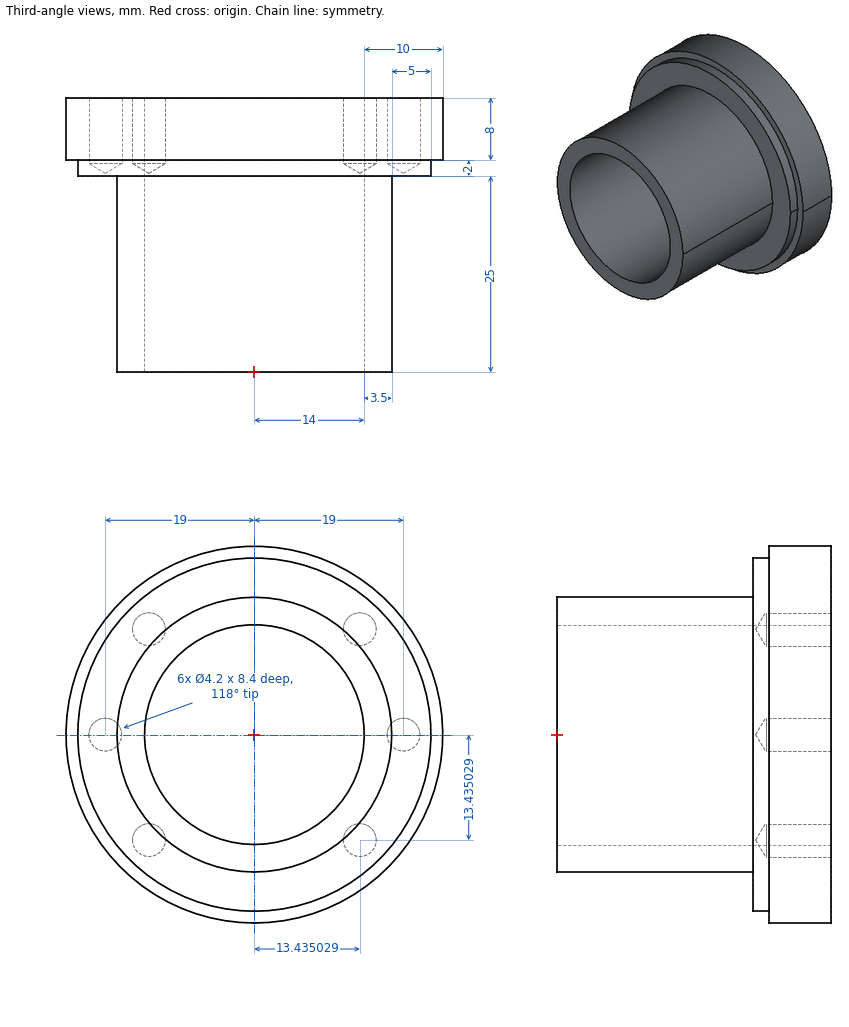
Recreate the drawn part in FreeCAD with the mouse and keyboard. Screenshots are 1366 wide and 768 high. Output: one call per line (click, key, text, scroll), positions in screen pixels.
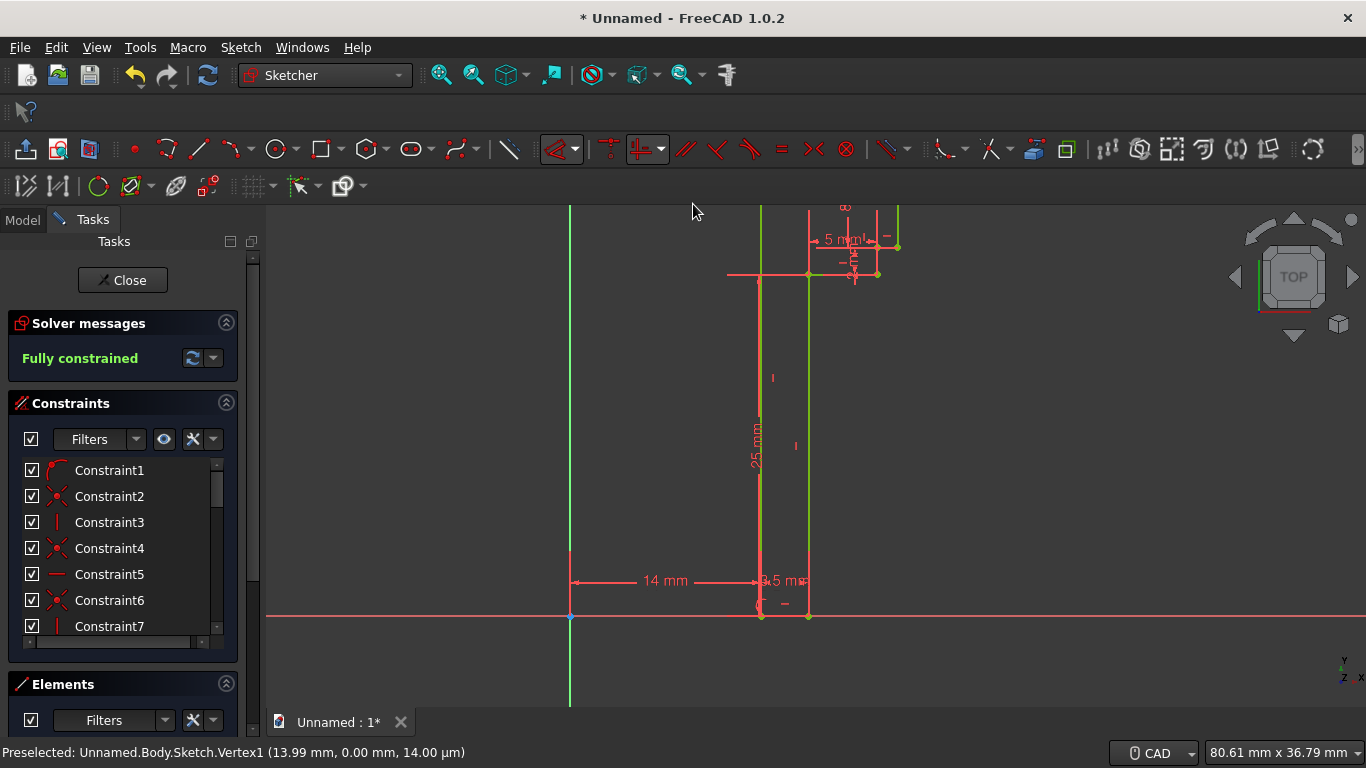
click(123, 280)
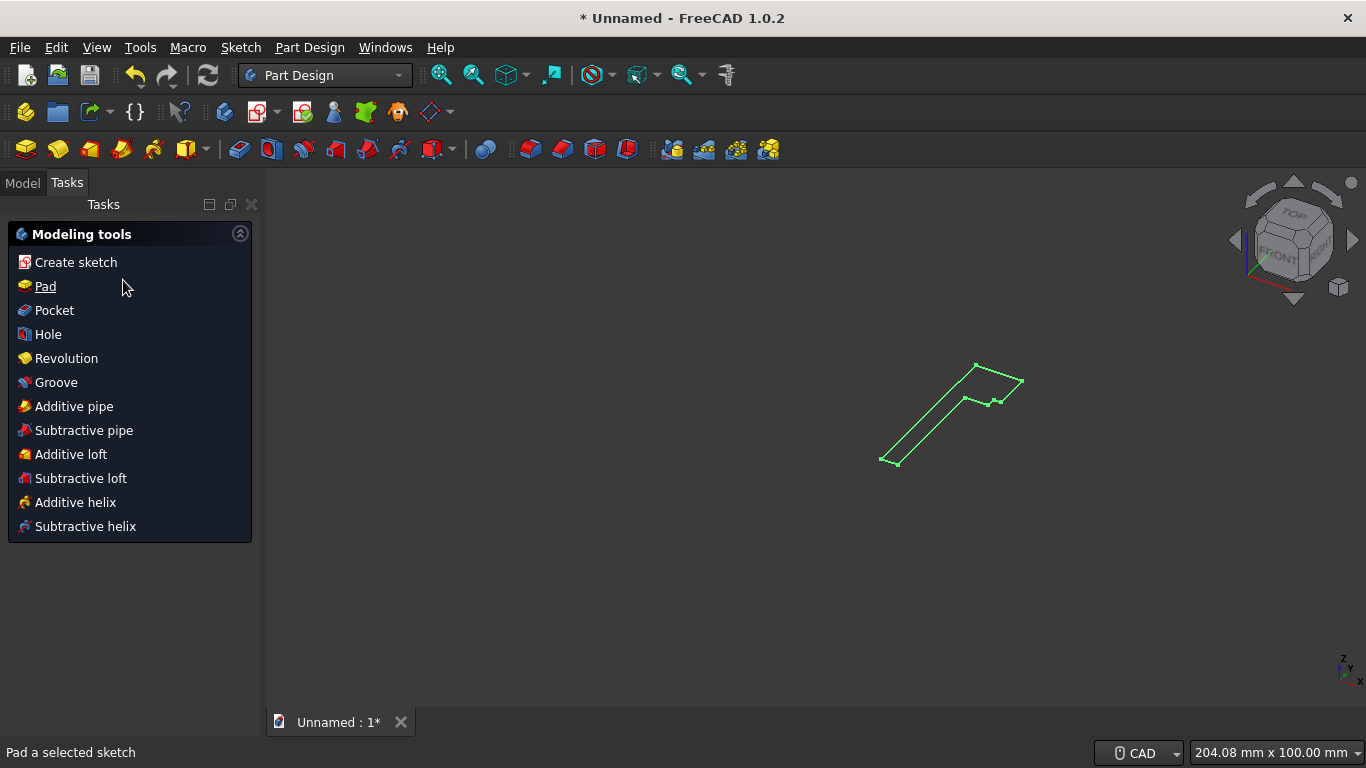
click(58, 150)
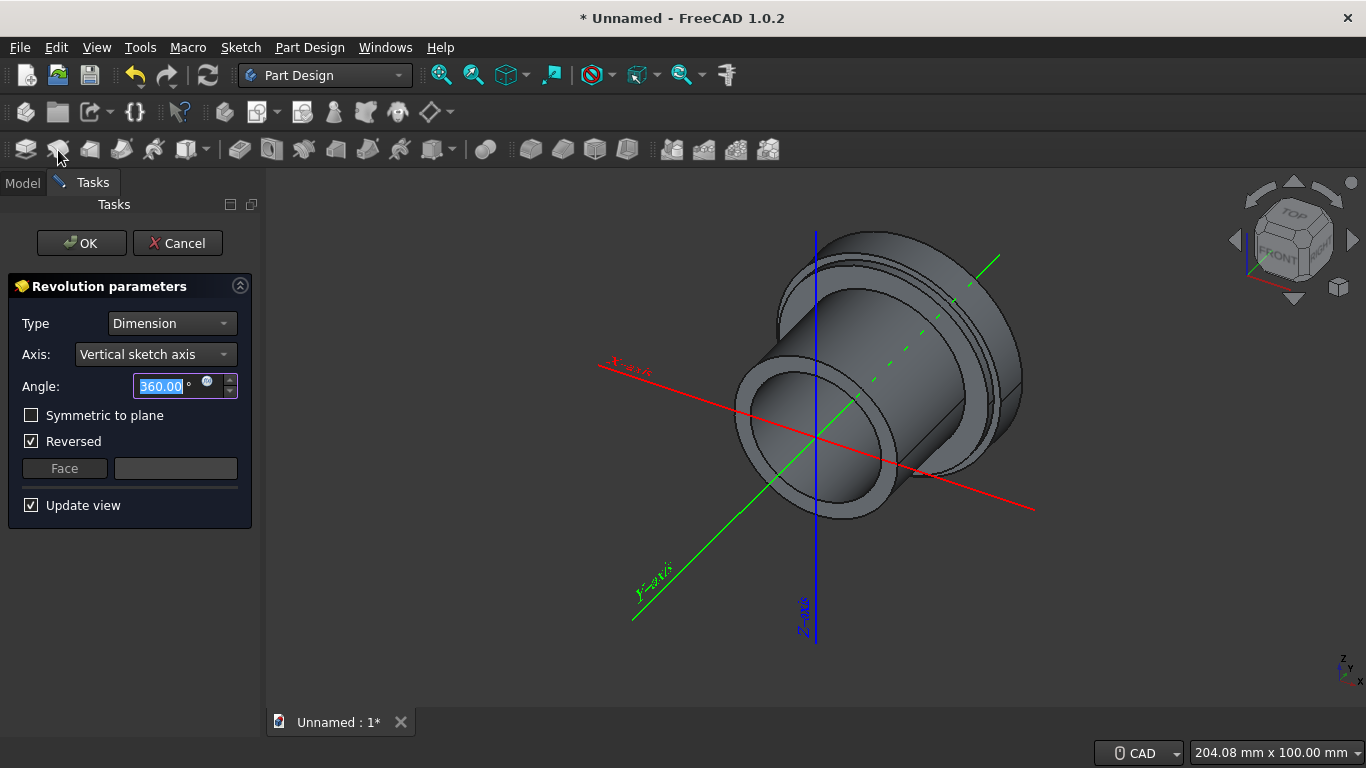
click(82, 243)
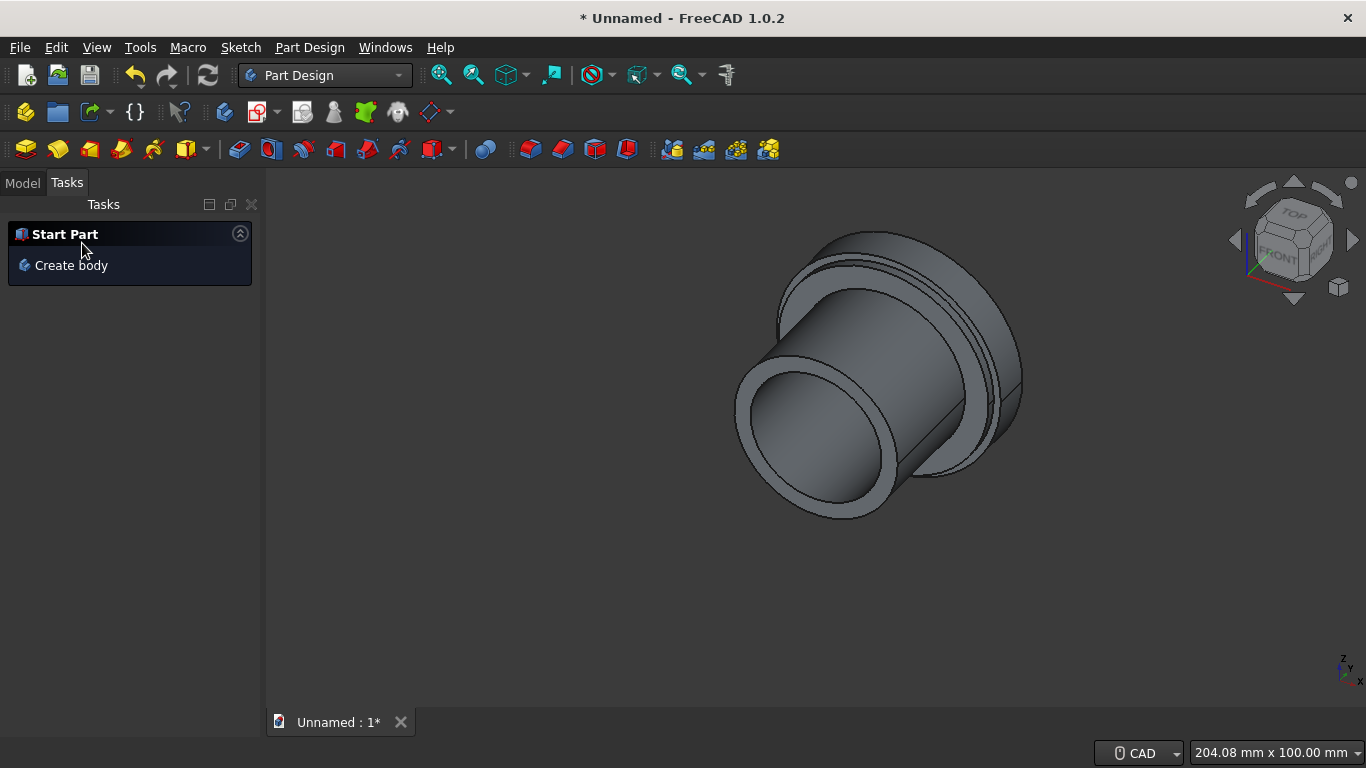
key(4)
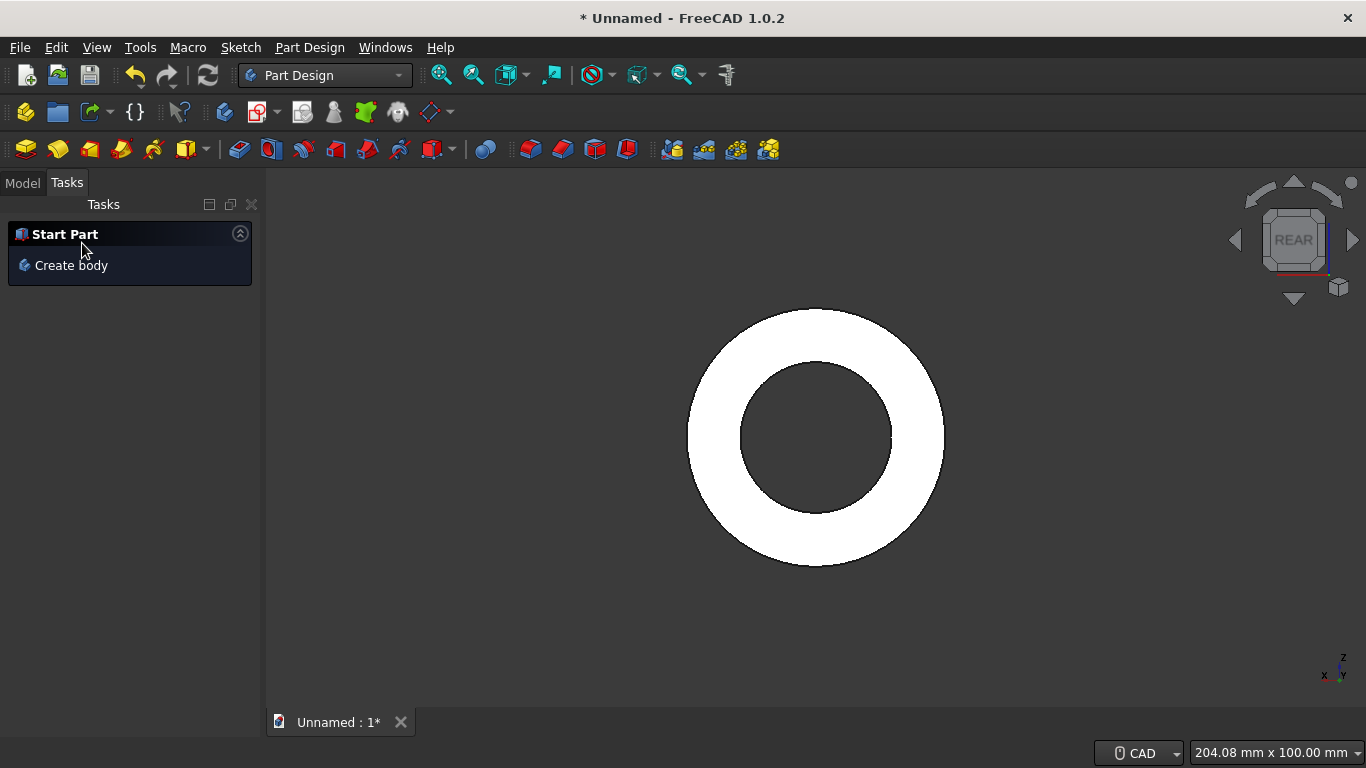
click(890, 510)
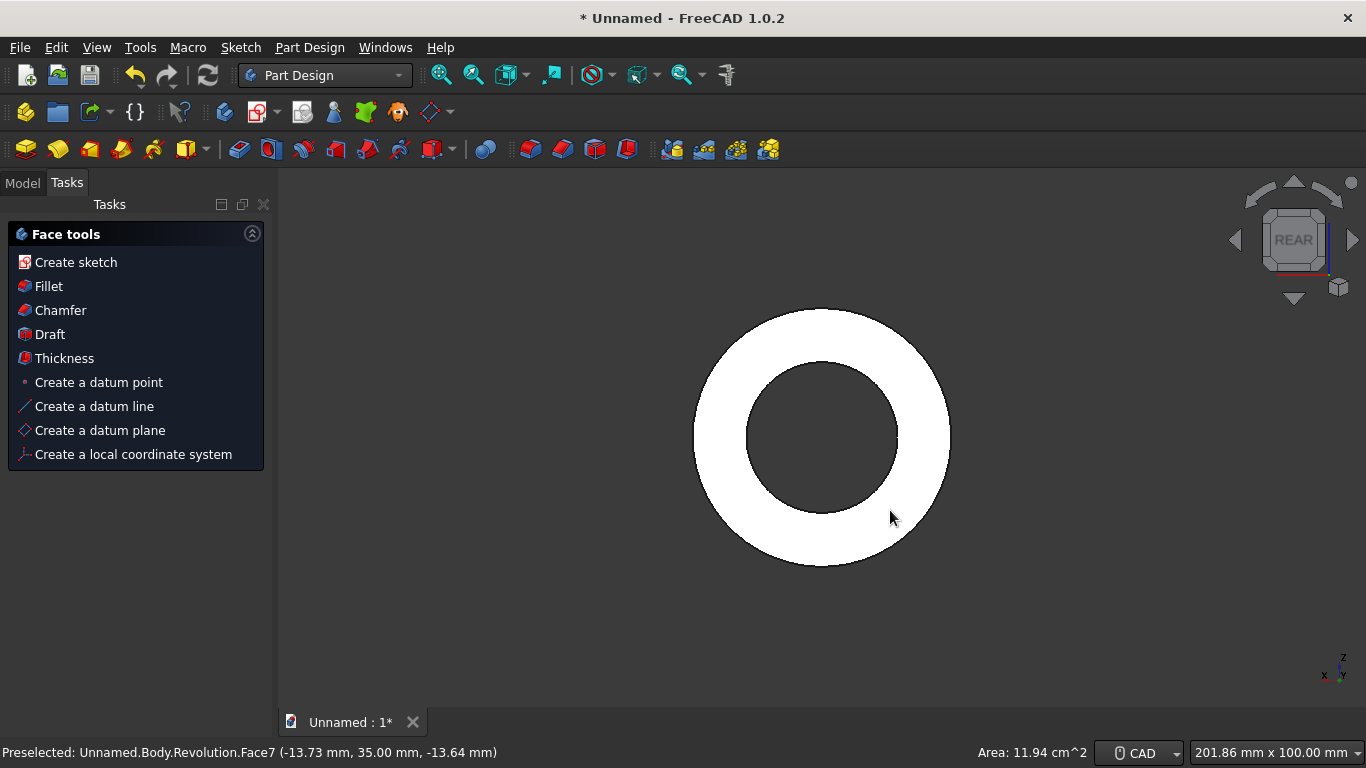
click(258, 112)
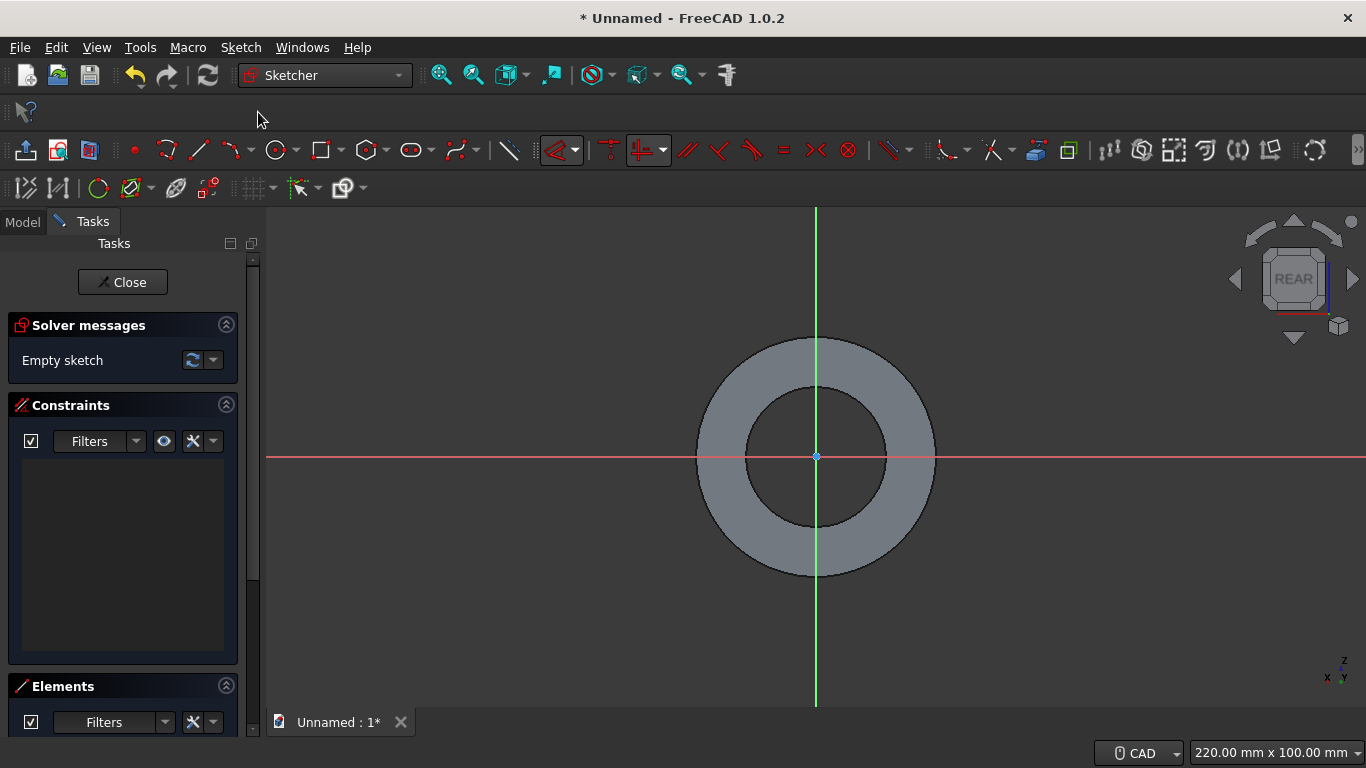
scroll(872, 457, up, 4)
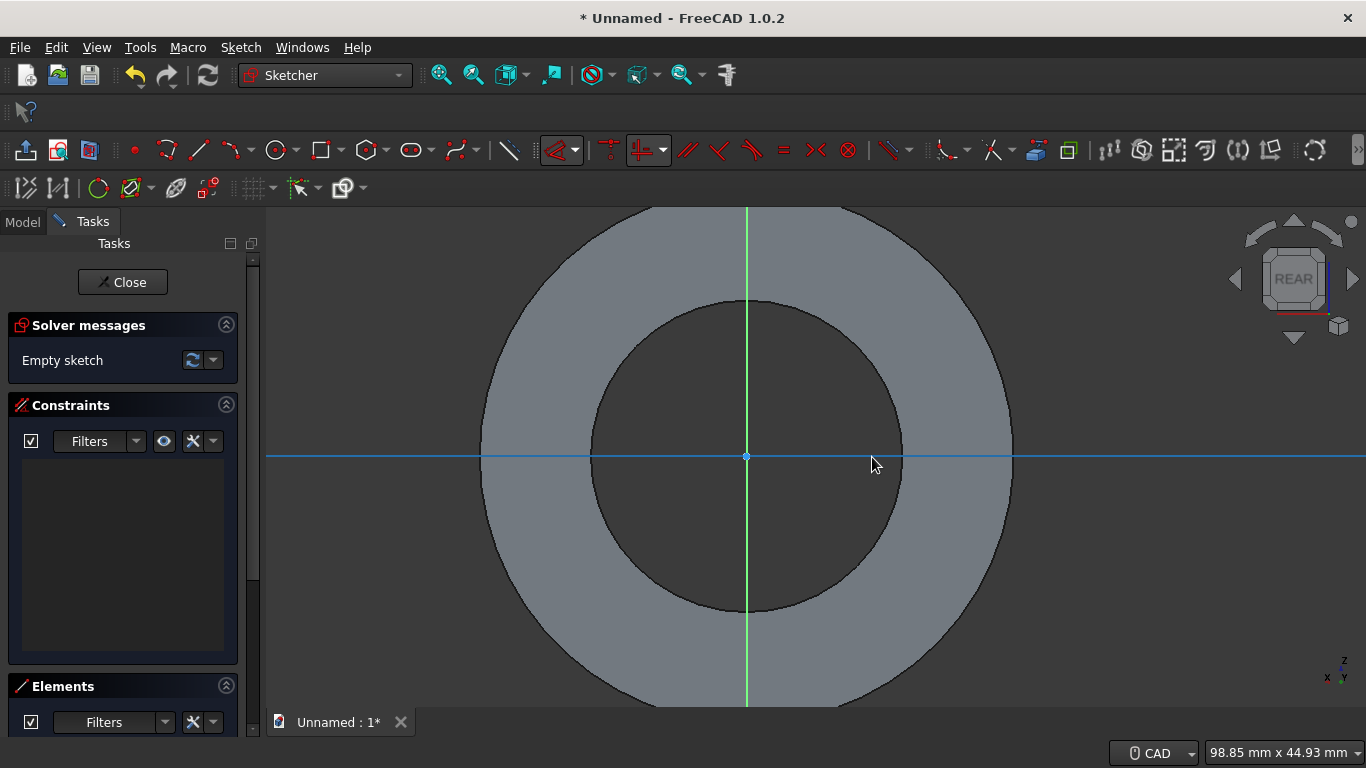
click(276, 150)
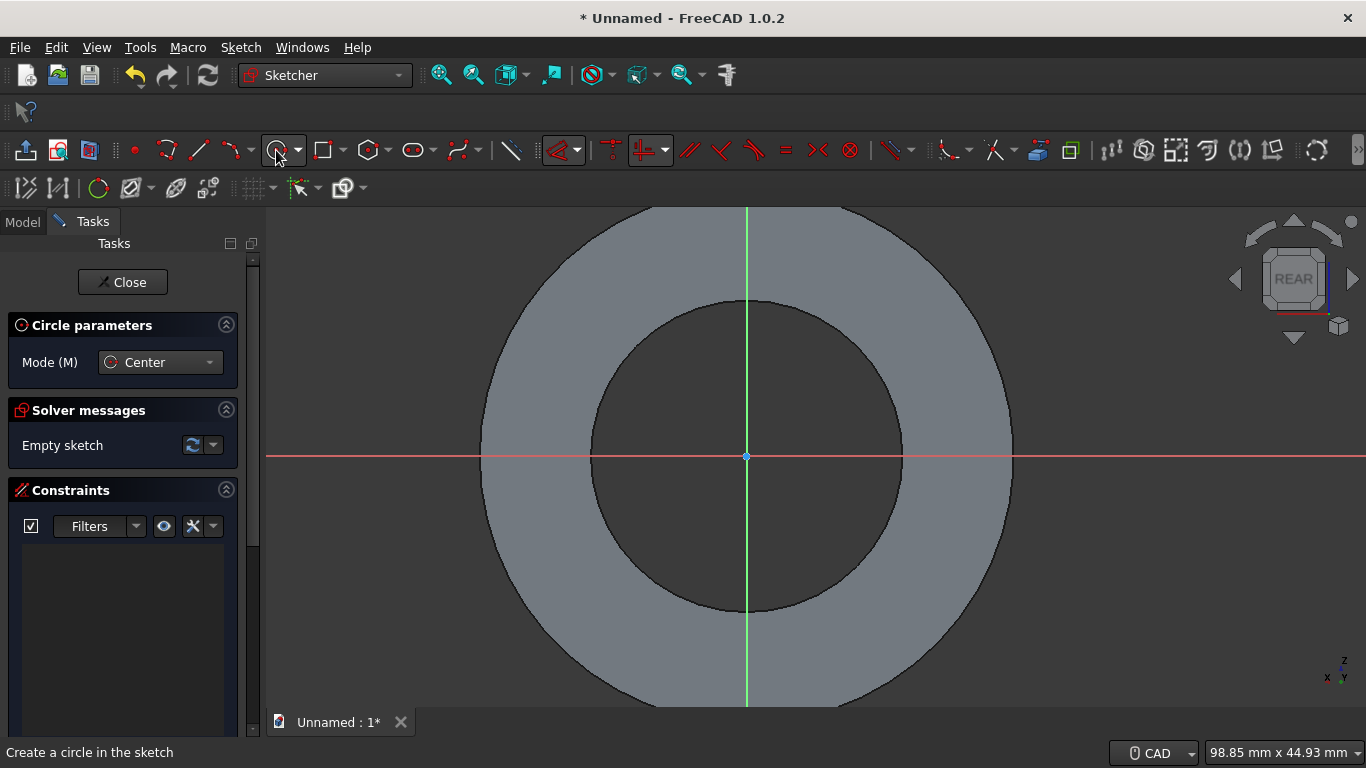
click(958, 456)
click(975, 440)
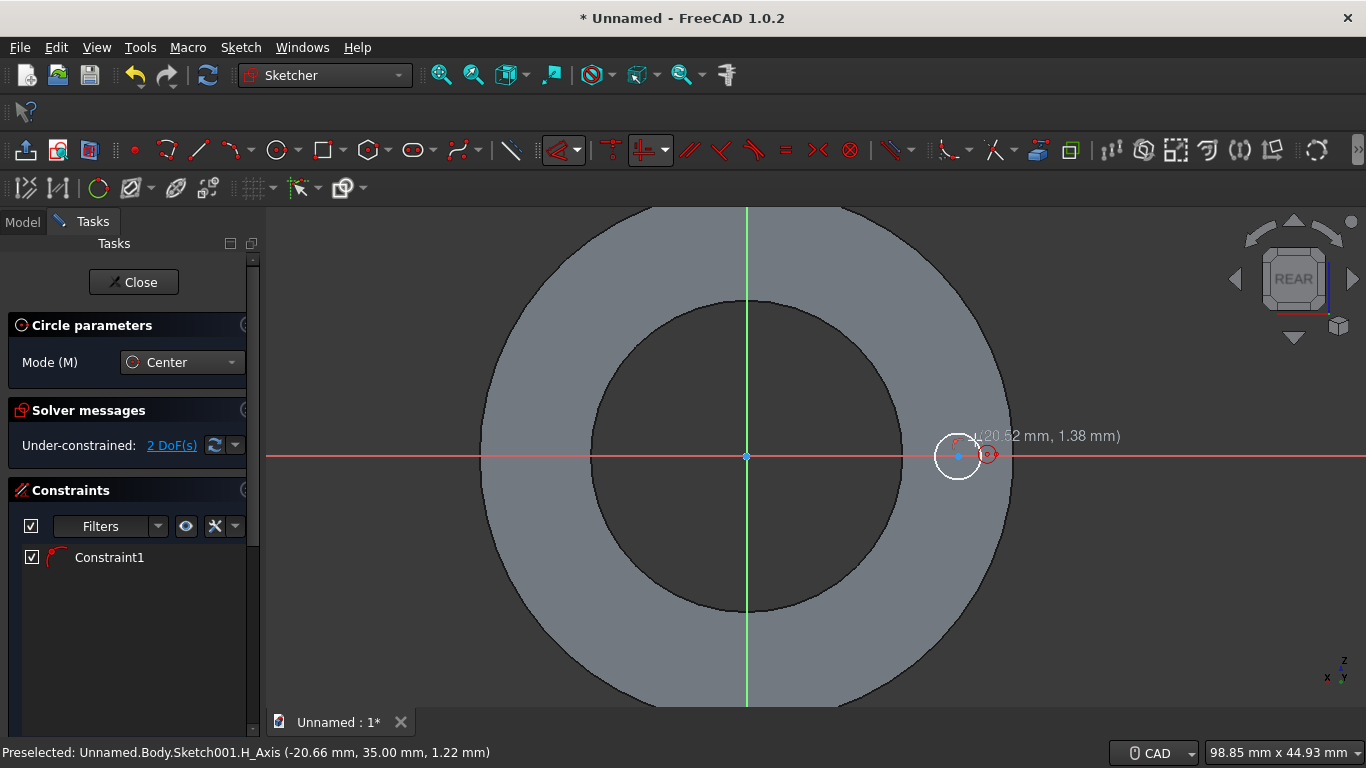
click(535, 456)
click(552, 440)